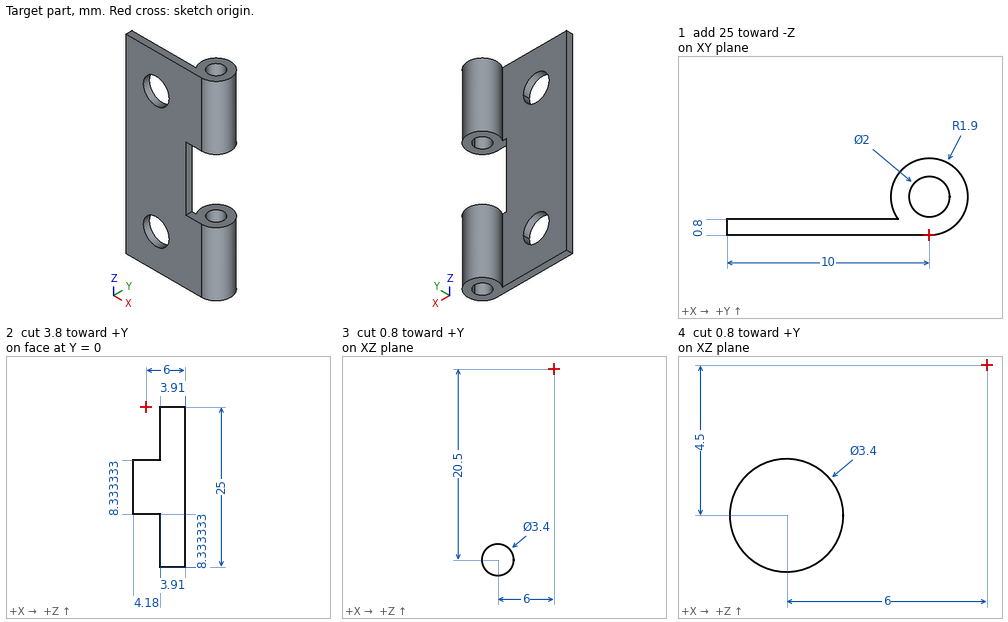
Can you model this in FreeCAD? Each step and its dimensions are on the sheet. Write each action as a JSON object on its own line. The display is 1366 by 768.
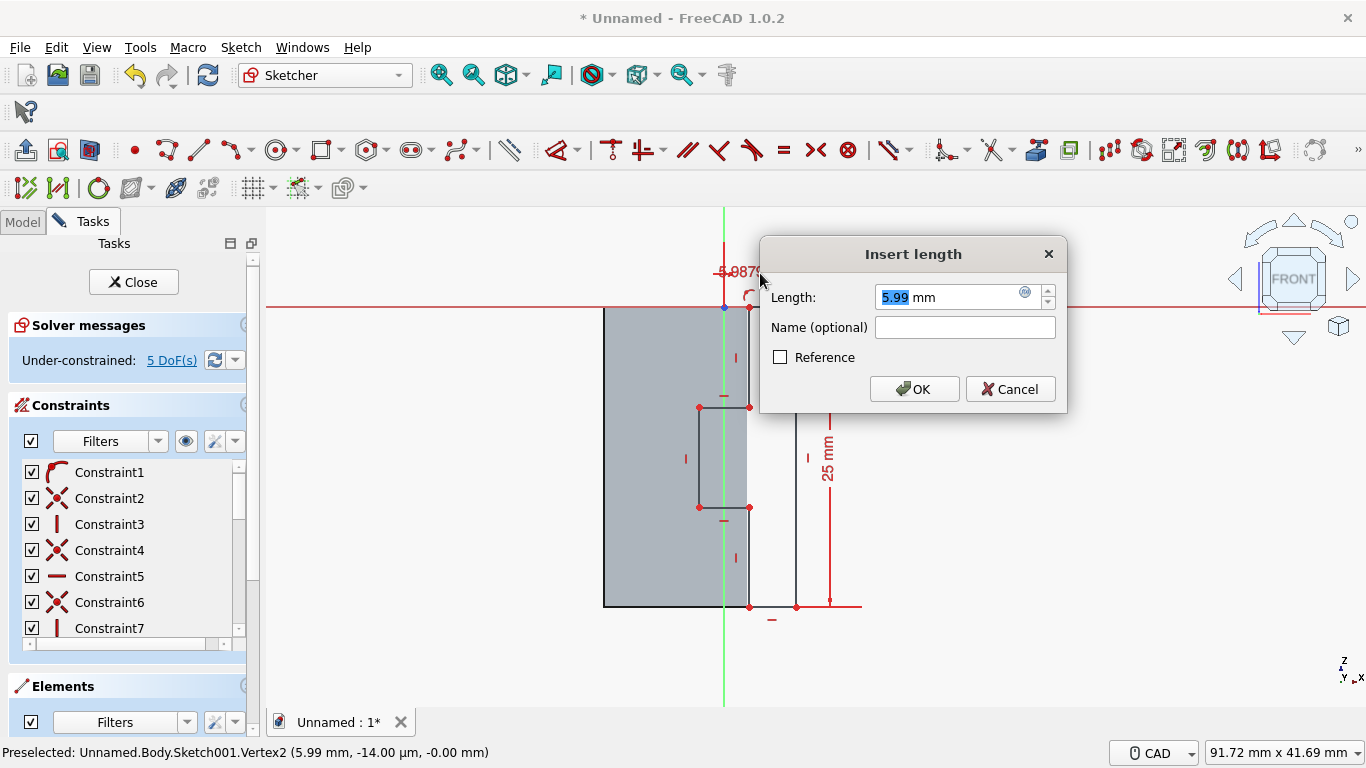
{"action": "type", "text": "6"}
{"action": "key", "text": "Return"}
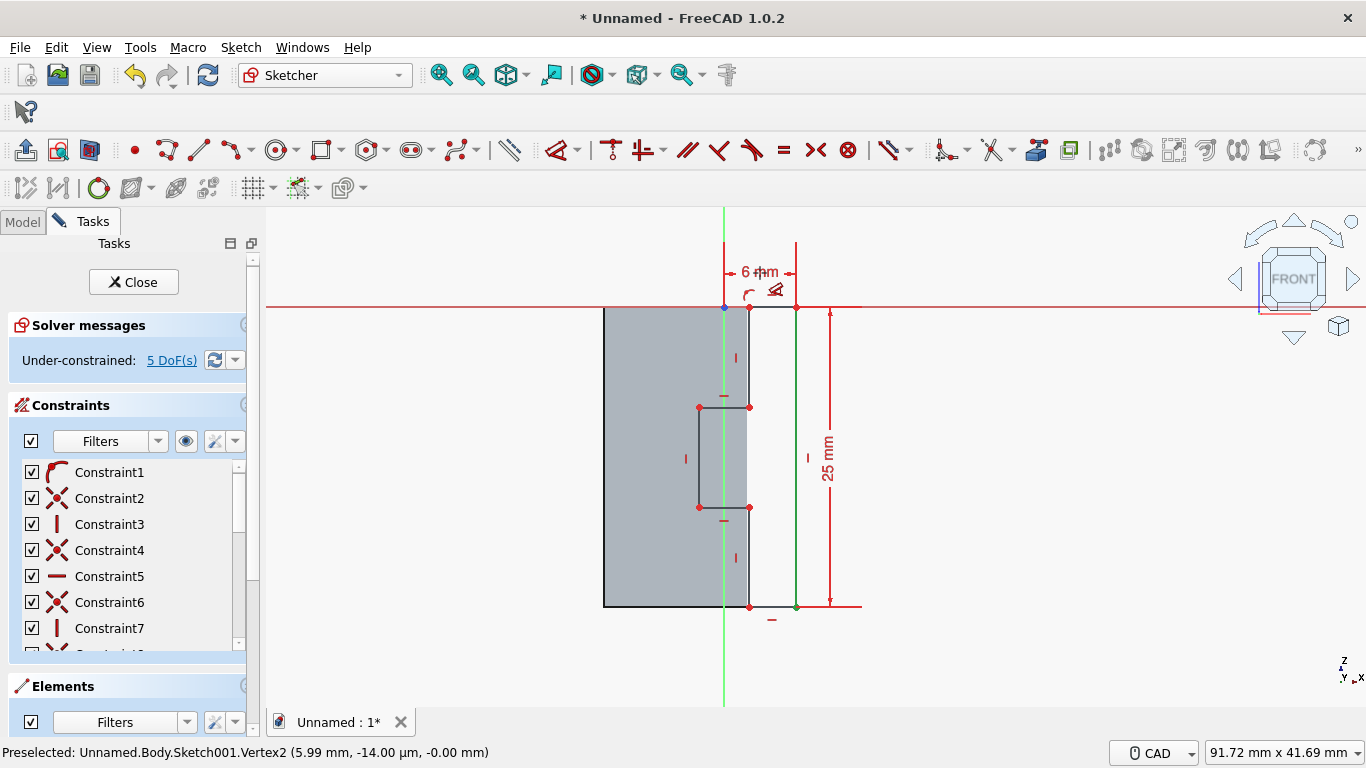
{"action": "left_click", "coordinate": [763, 307]}
{"action": "left_click", "coordinate": [773, 341]}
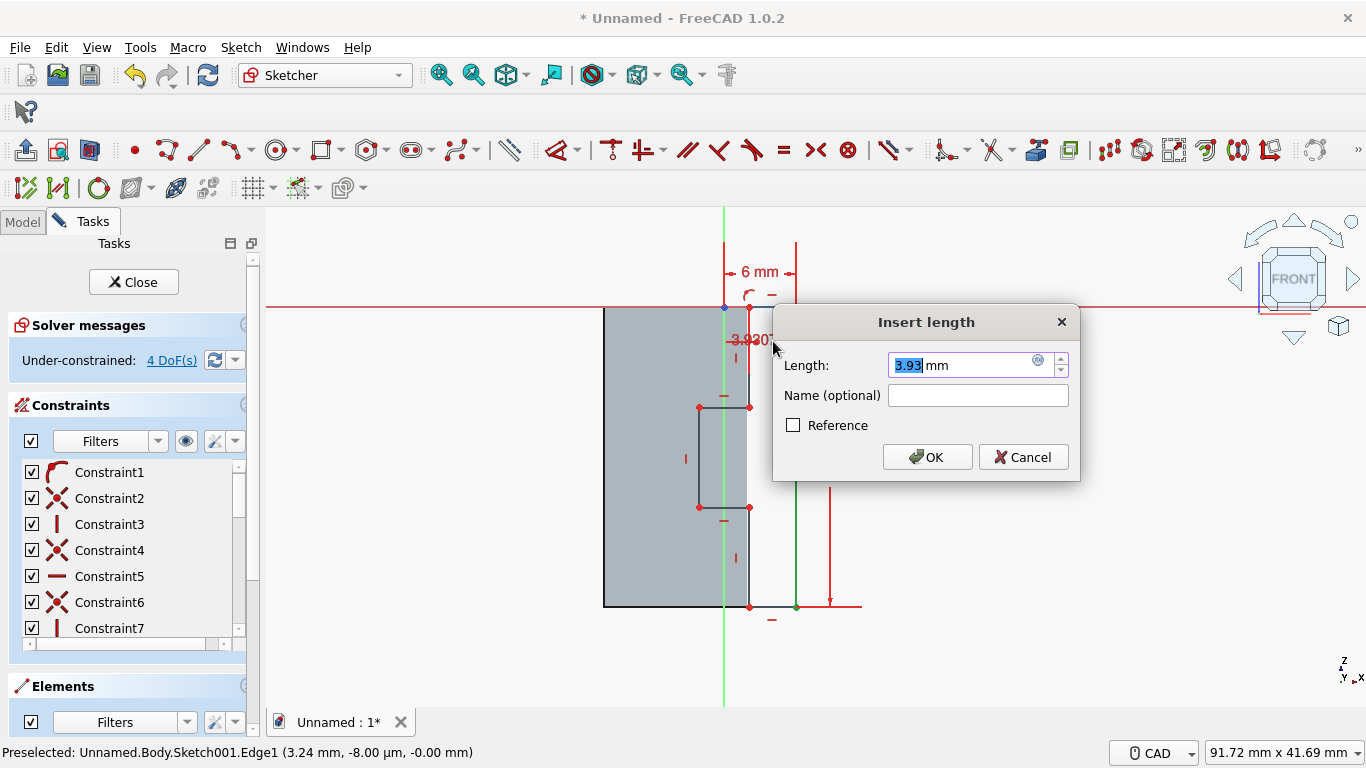
{"action": "type", "text": "3.91"}
{"action": "key", "text": "Return"}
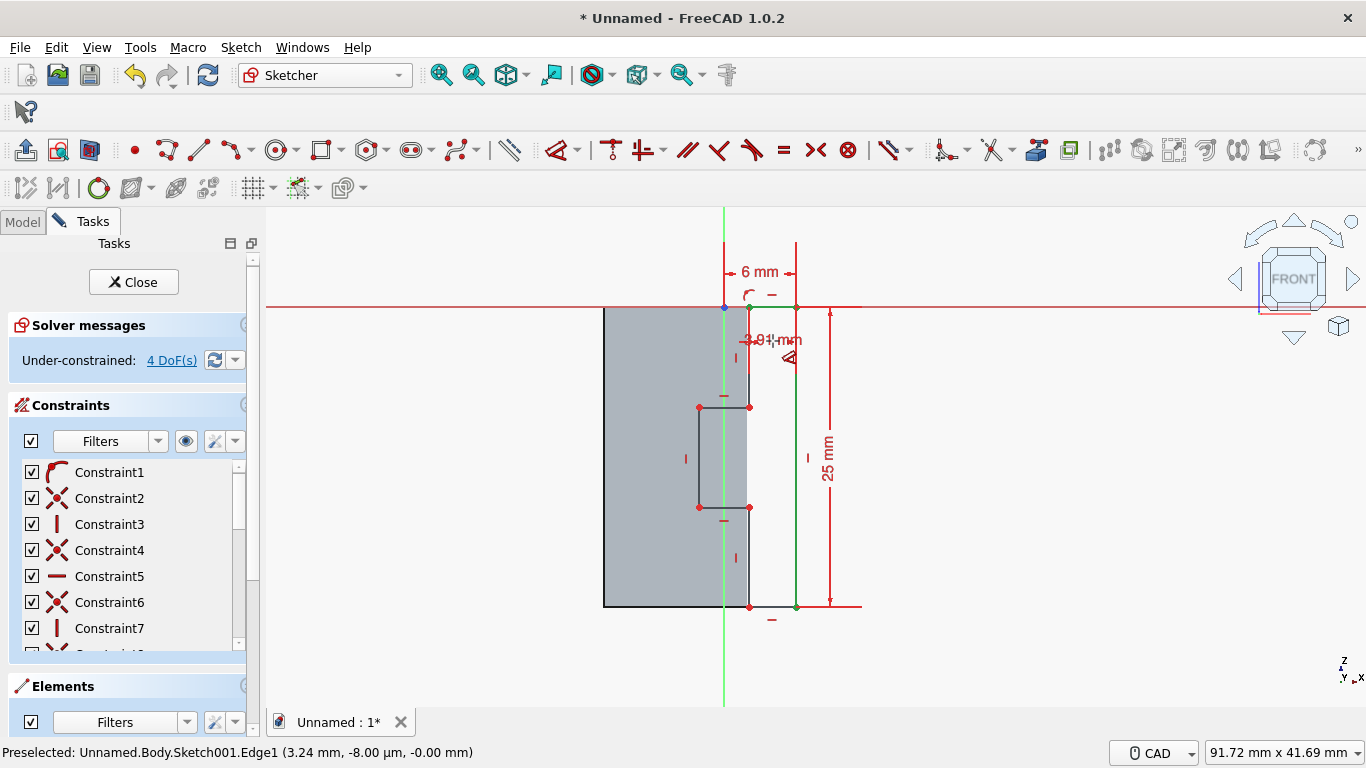
{"action": "left_click", "coordinate": [782, 607]}
{"action": "left_click", "coordinate": [773, 641]}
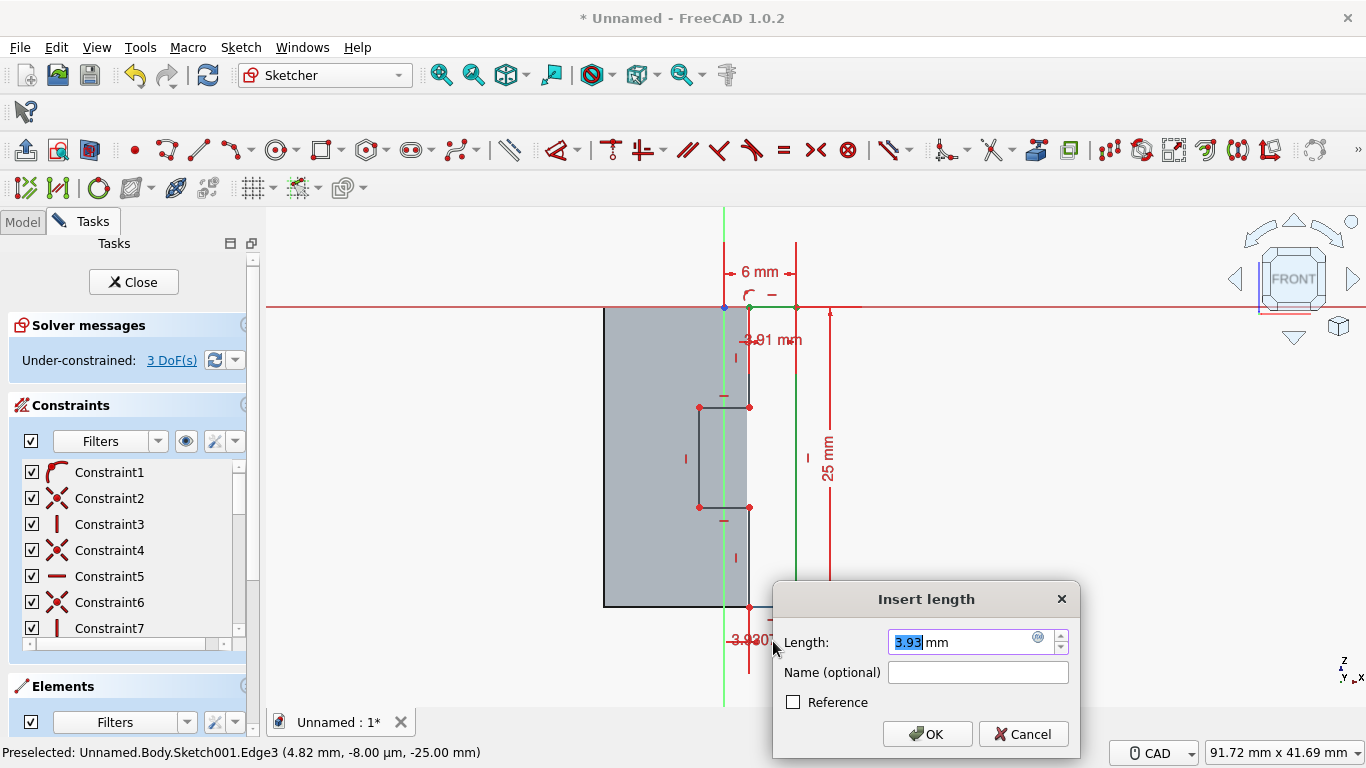
{"action": "type", "text": "3.91"}
{"action": "key", "text": "Return"}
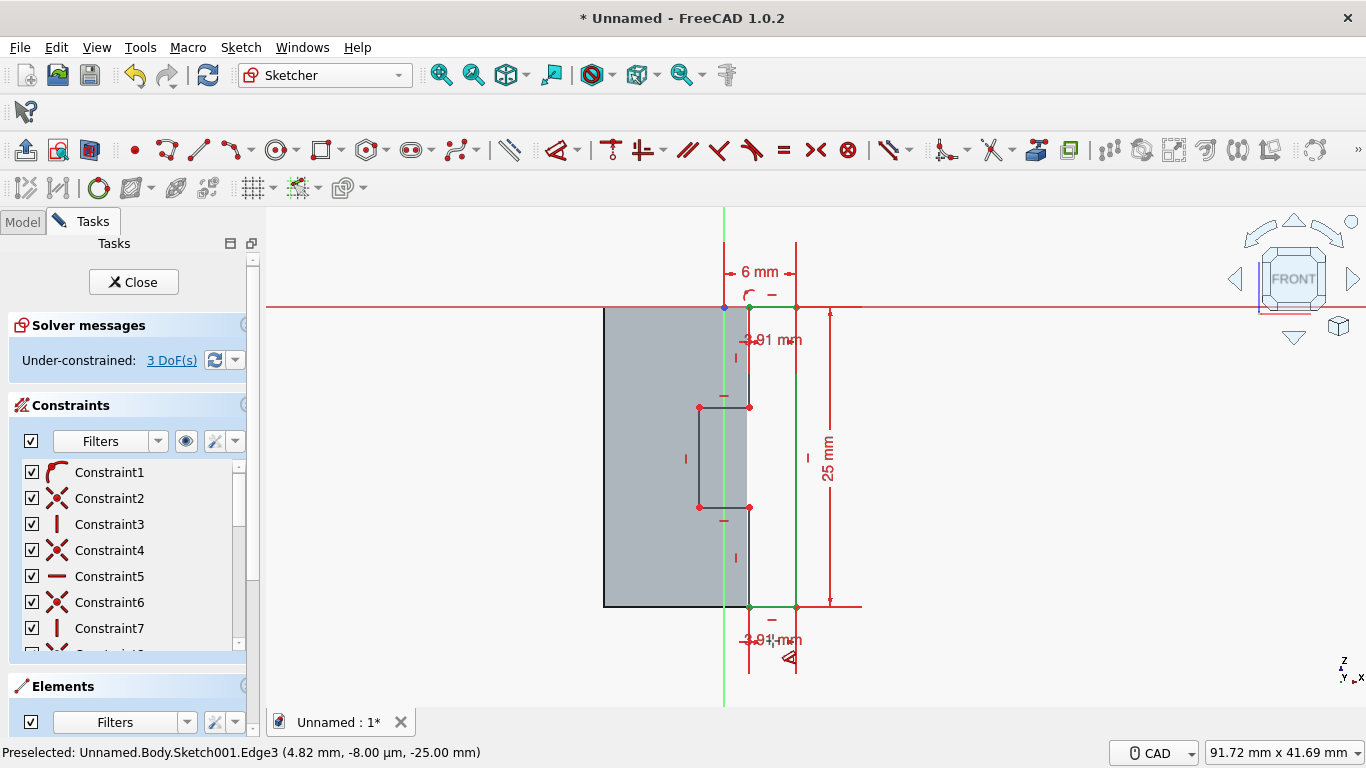
{"action": "scroll", "coordinate": [734, 508], "scroll_direction": "up", "scroll_amount": 2}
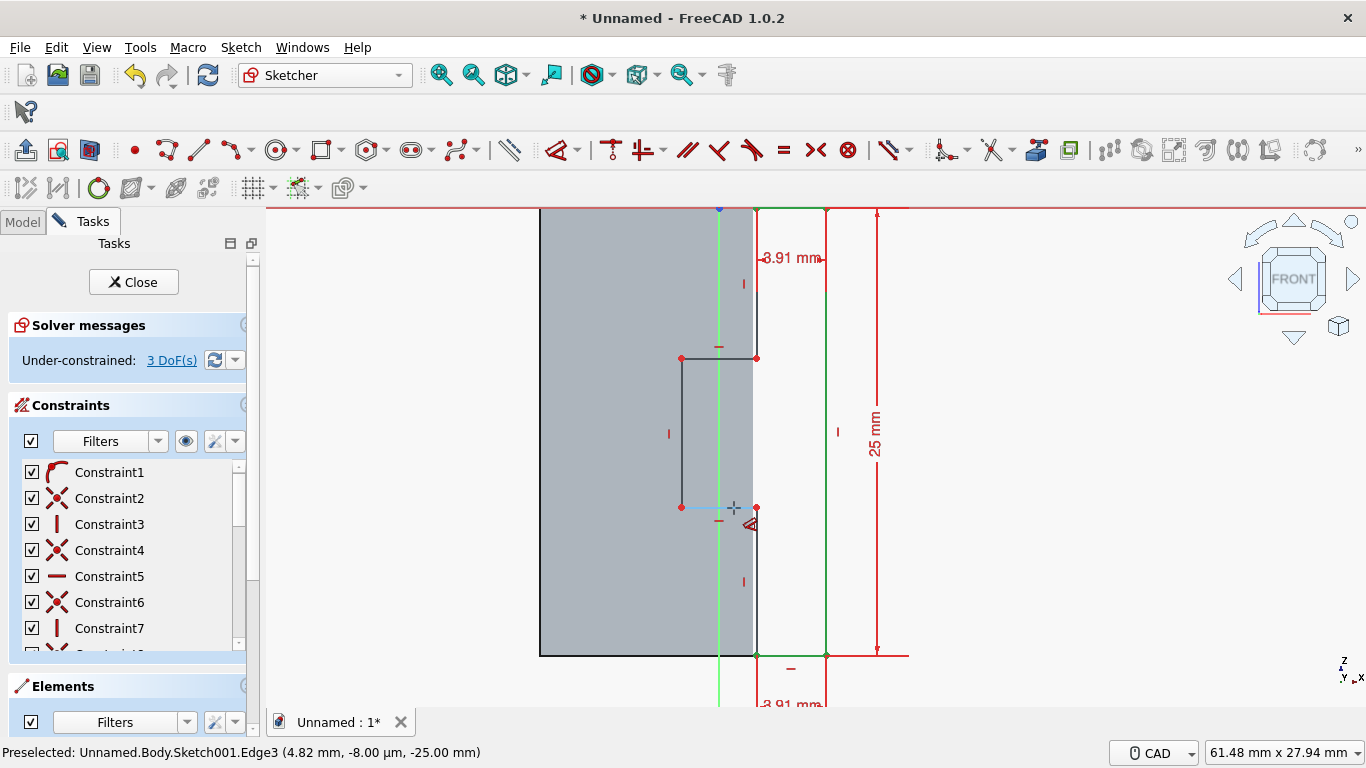
{"action": "left_click", "coordinate": [734, 508]}
{"action": "left_click", "coordinate": [702, 542]}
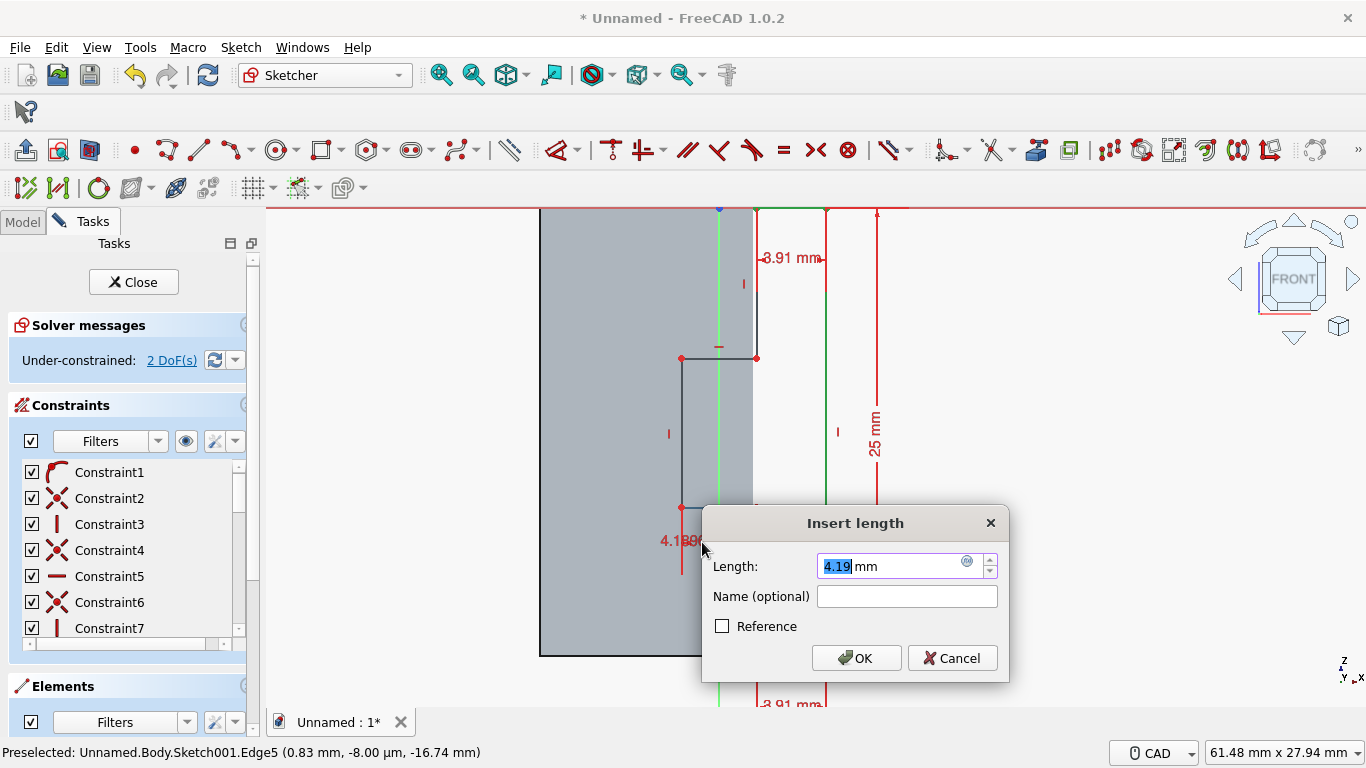
{"action": "type", "text": "4.18"}
{"action": "key", "text": "Return"}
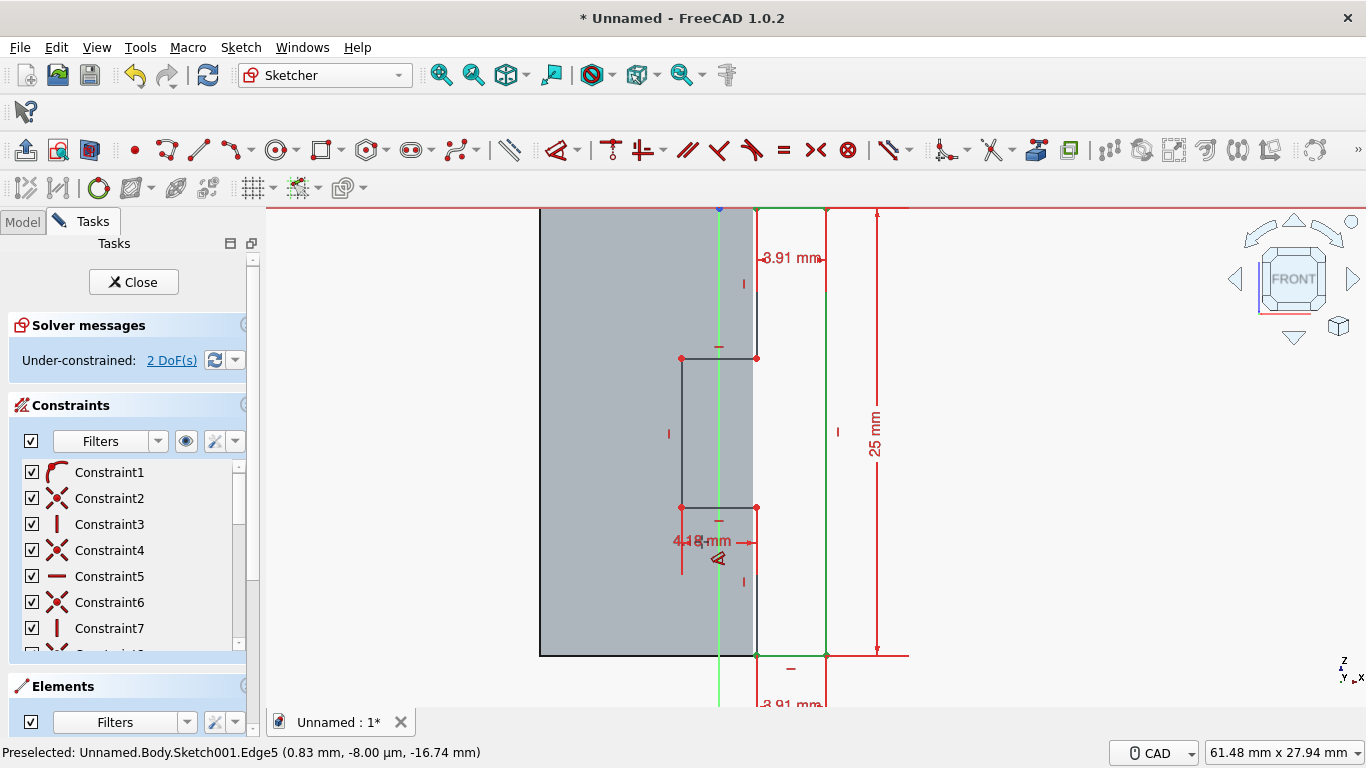
{"action": "left_click", "coordinate": [757, 611]}
{"action": "left_click", "coordinate": [791, 582]}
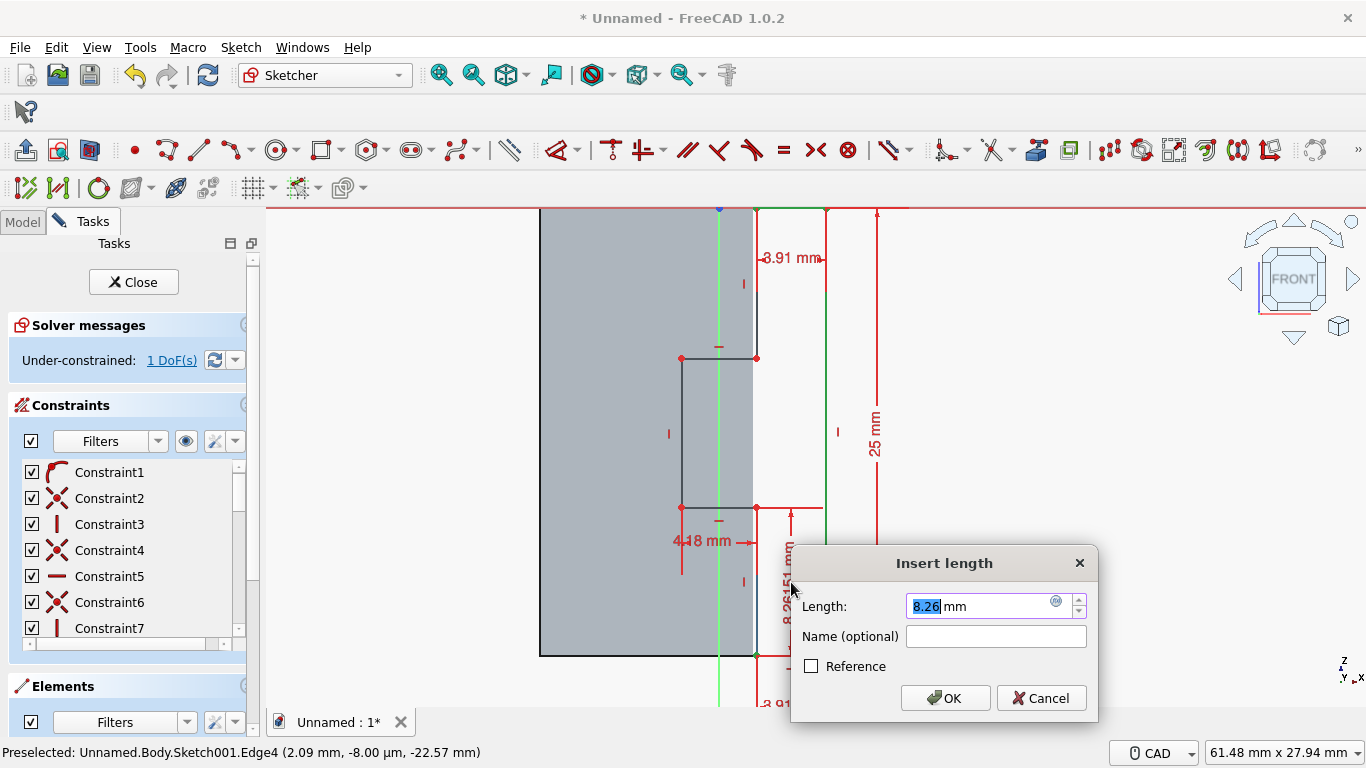
{"action": "type", "text": "8.333333"}
{"action": "key", "text": "Return"}